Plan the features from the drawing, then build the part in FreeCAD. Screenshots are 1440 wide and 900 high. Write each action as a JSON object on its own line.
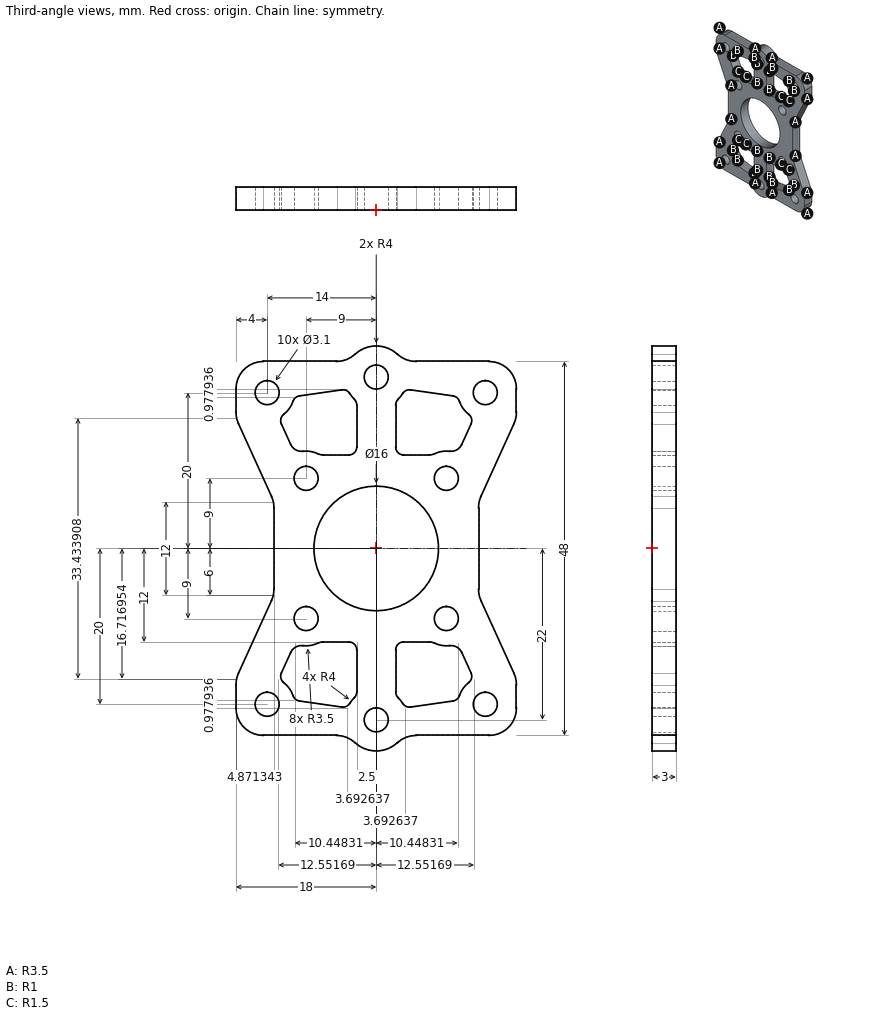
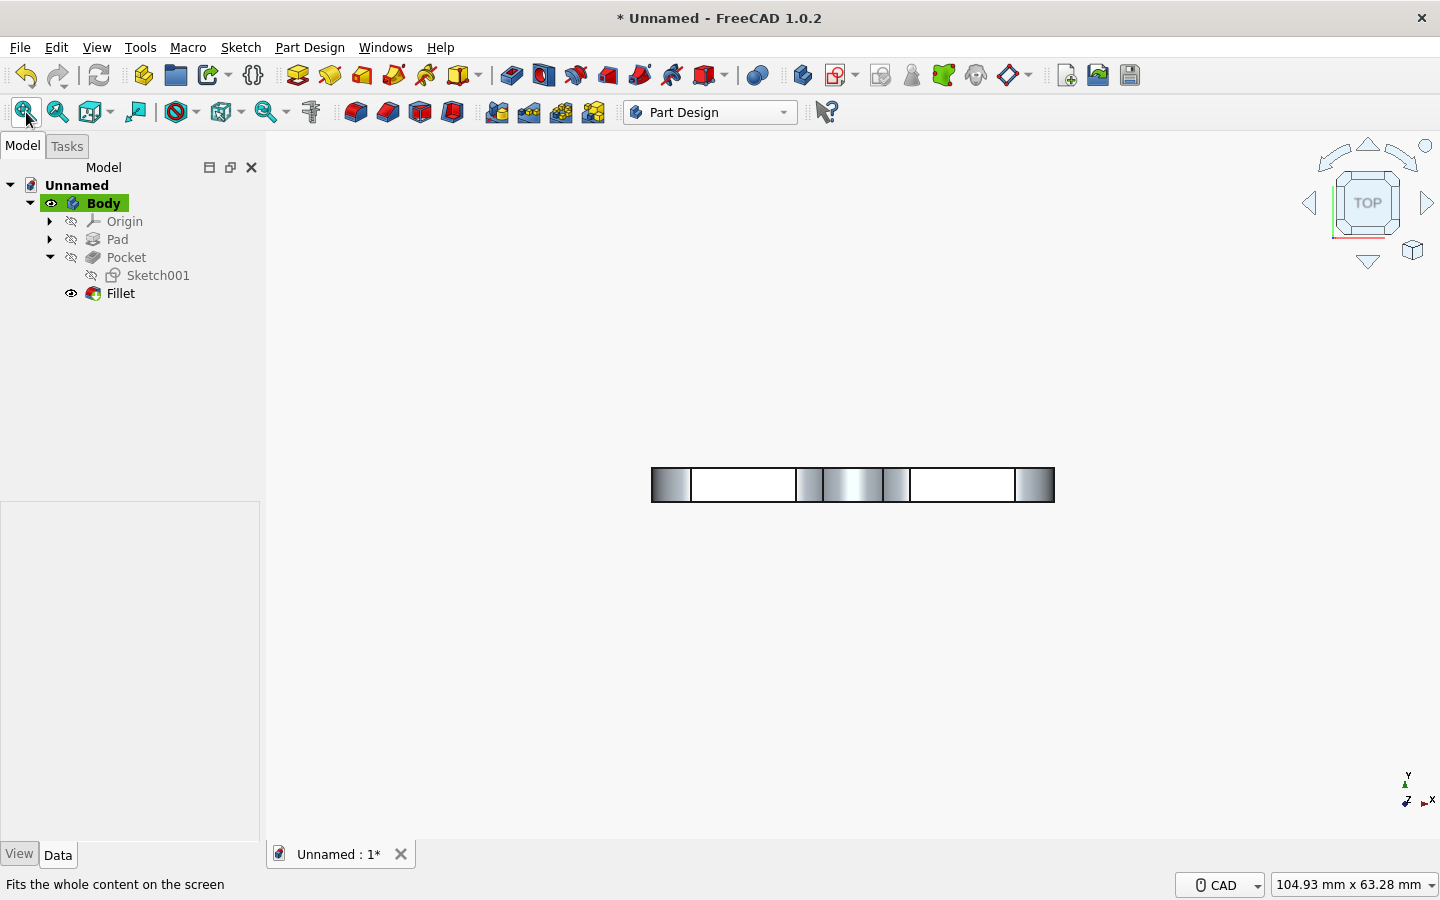
{"action": "left_click", "coordinate": [26, 112]}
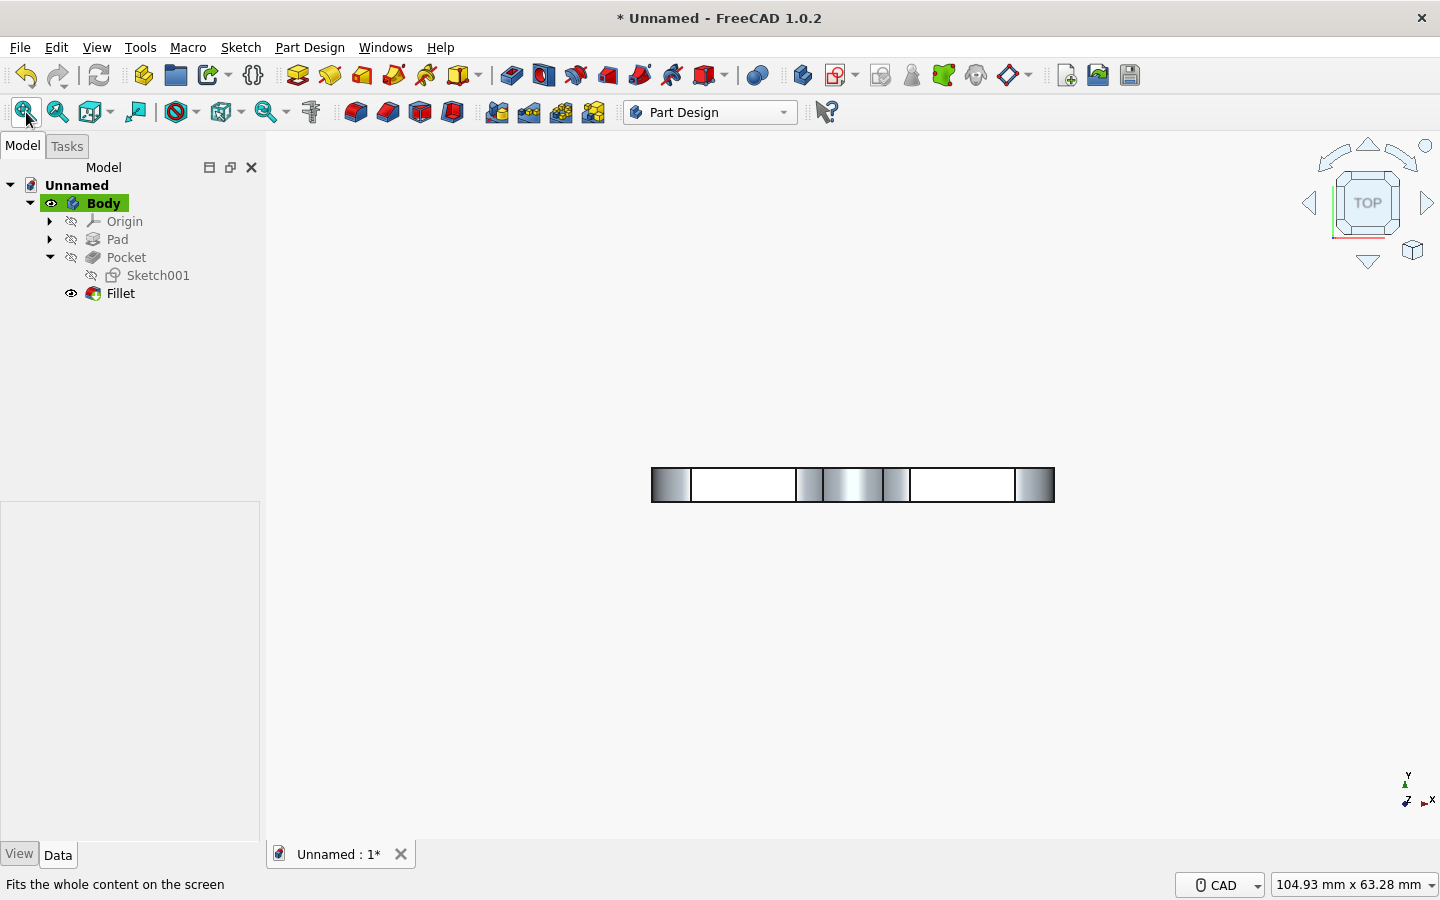
{"action": "key", "text": "1"}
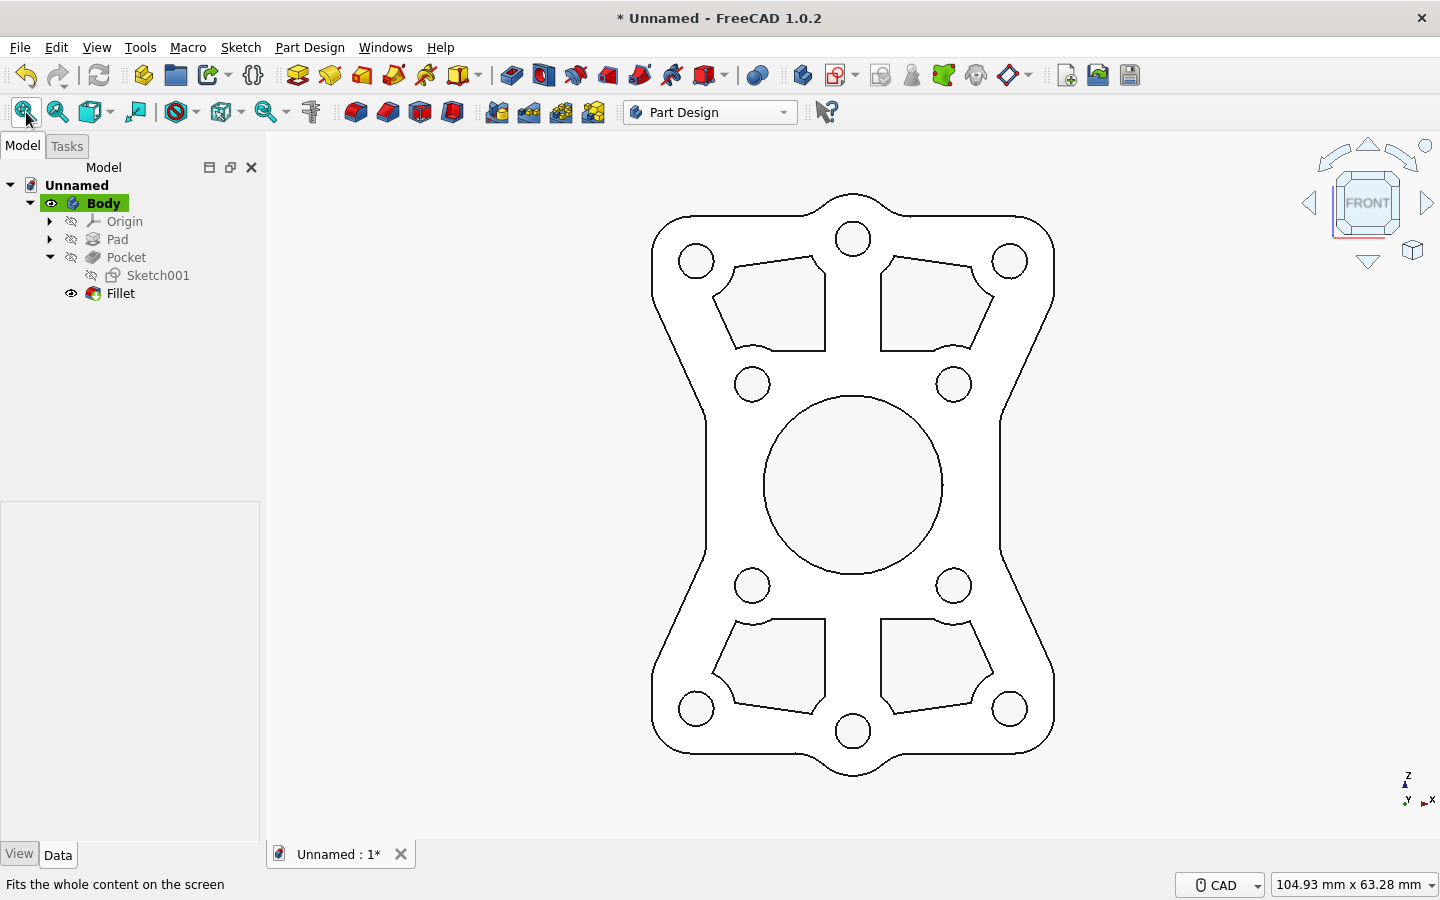
{"action": "key", "text": "3"}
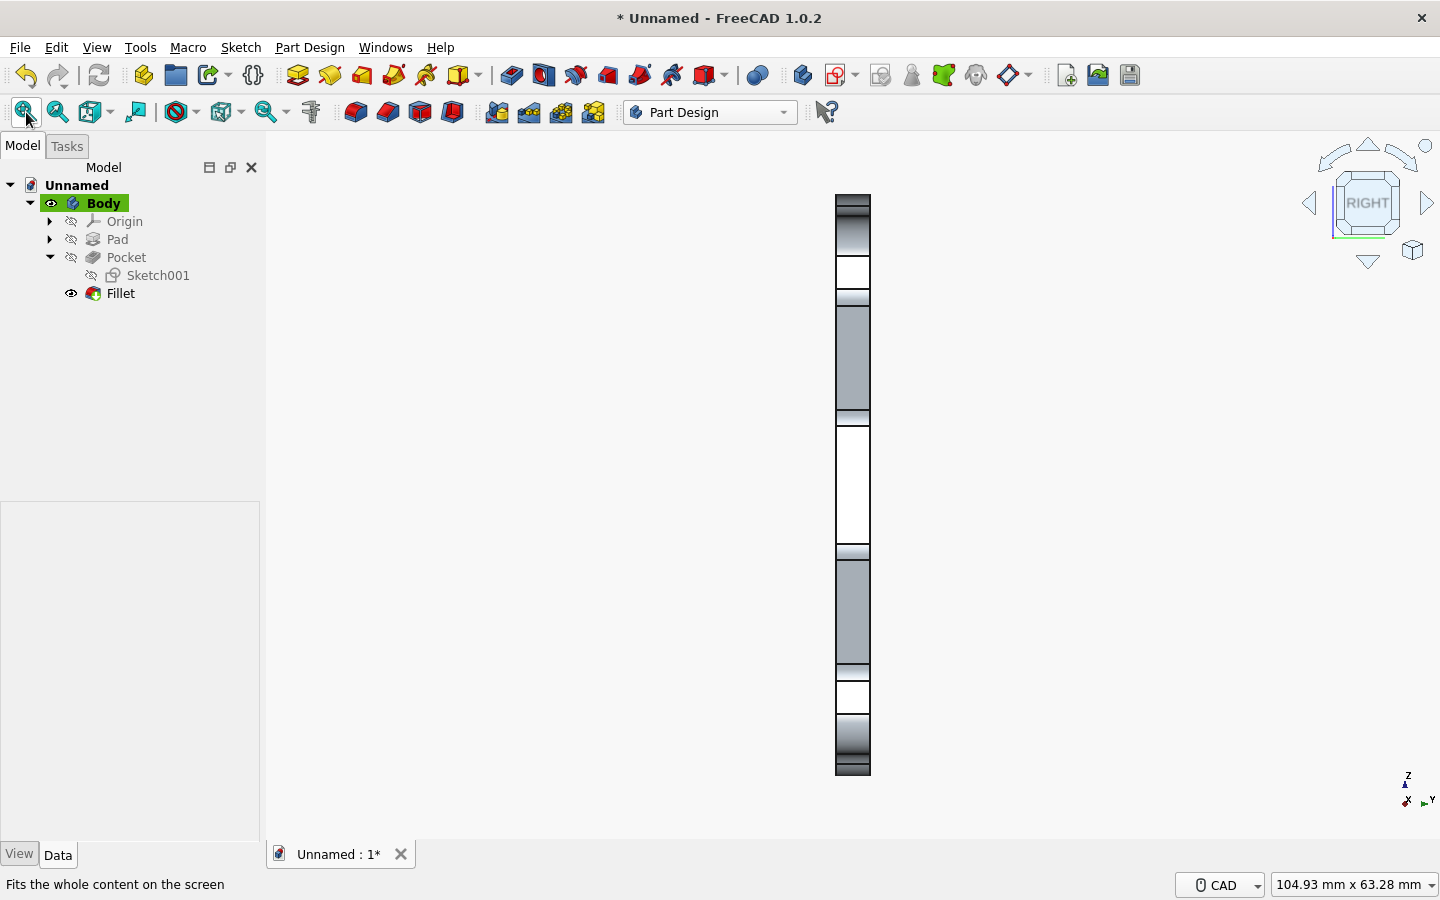
{"action": "key", "text": "5"}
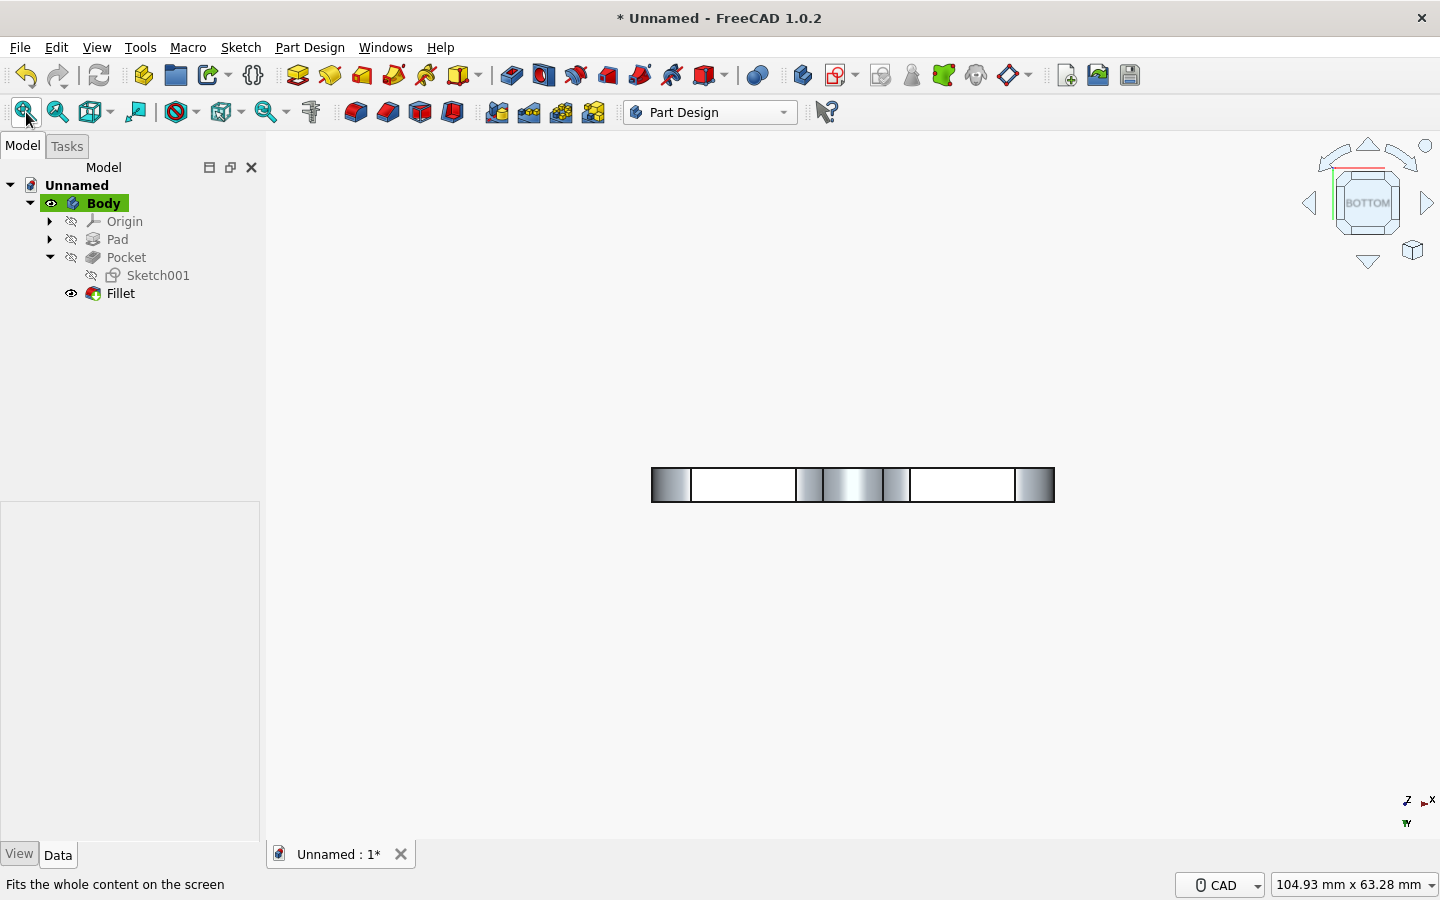
{"action": "left_click", "coordinate": [26, 112]}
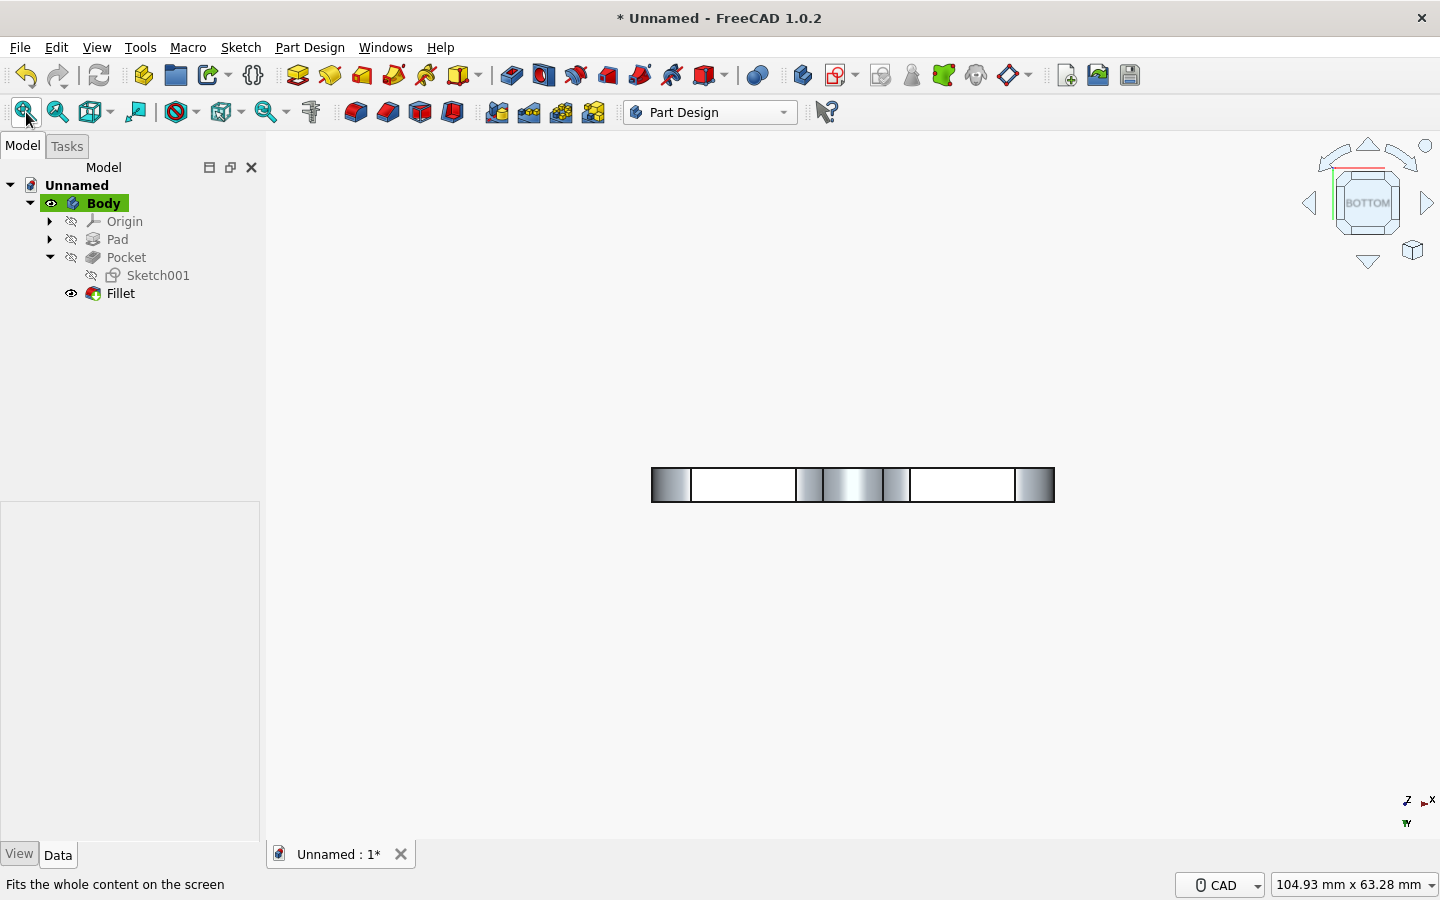
{"action": "key", "text": "4"}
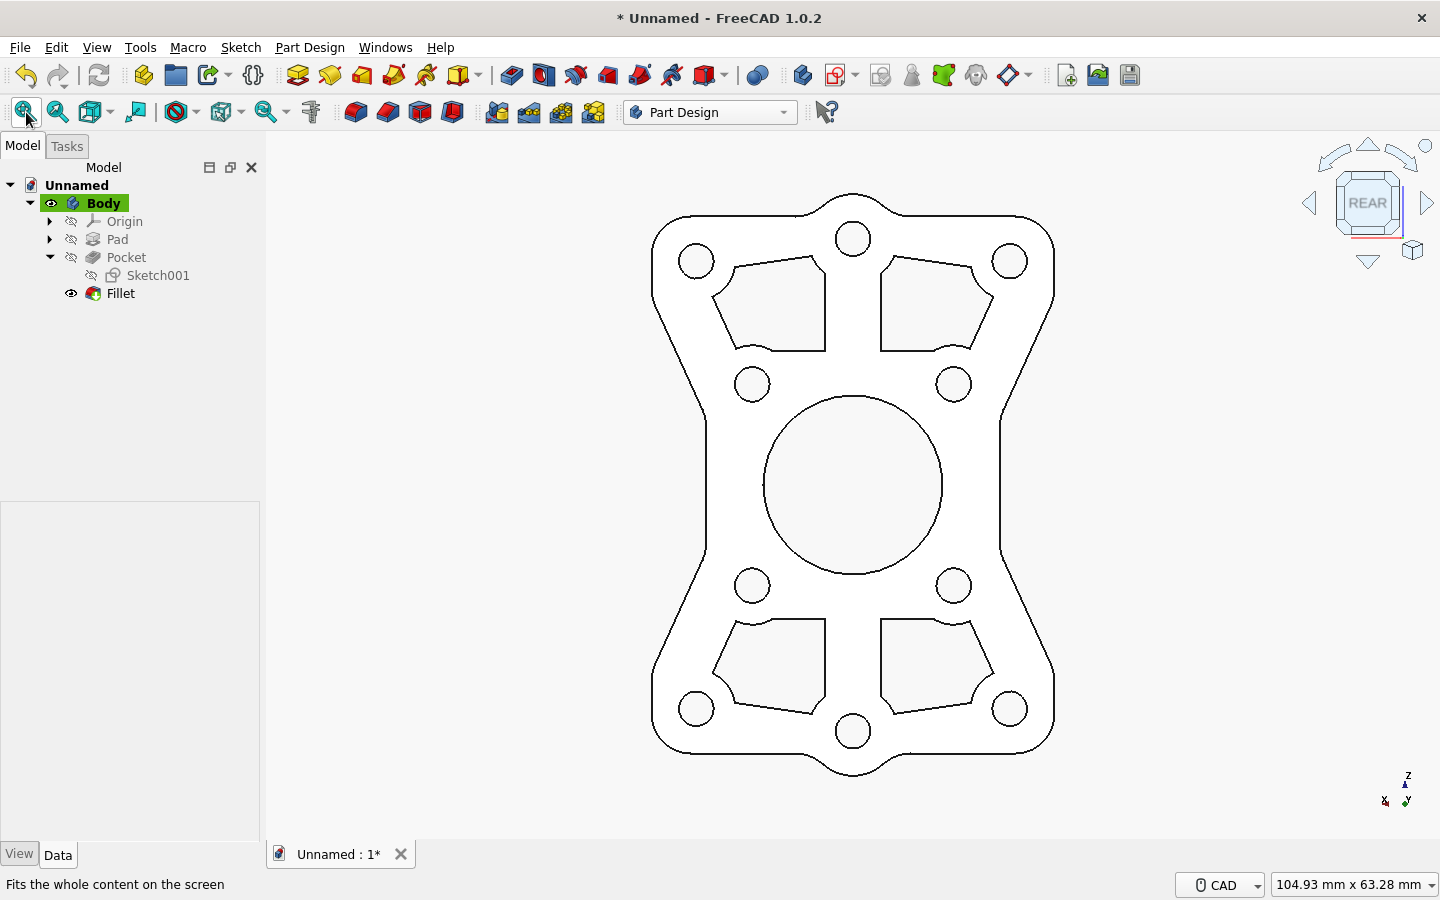
{"action": "key", "text": "6"}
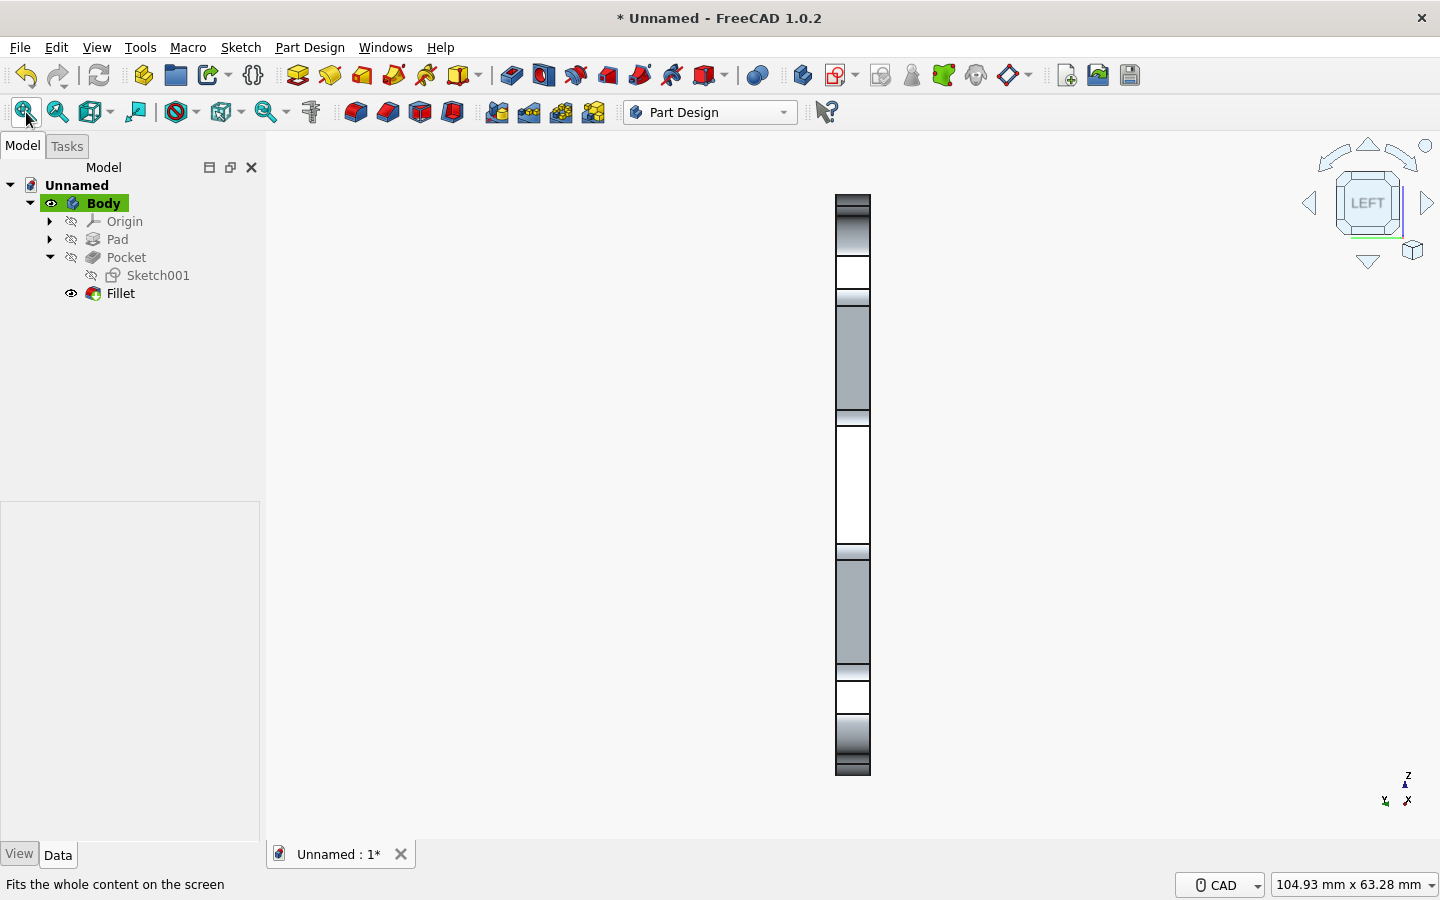
{"action": "key", "text": "v 3"}